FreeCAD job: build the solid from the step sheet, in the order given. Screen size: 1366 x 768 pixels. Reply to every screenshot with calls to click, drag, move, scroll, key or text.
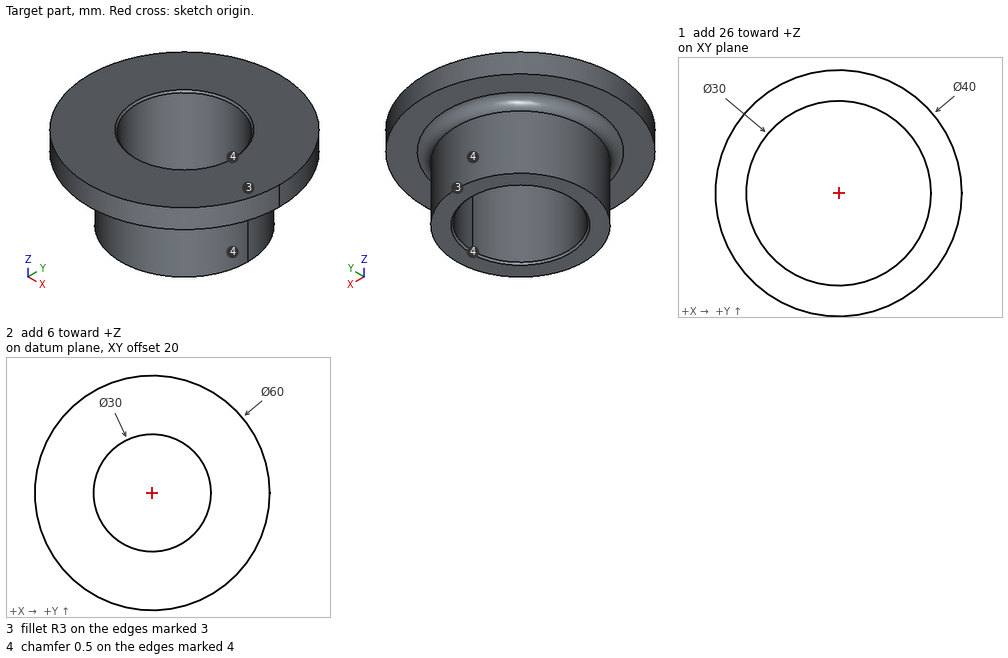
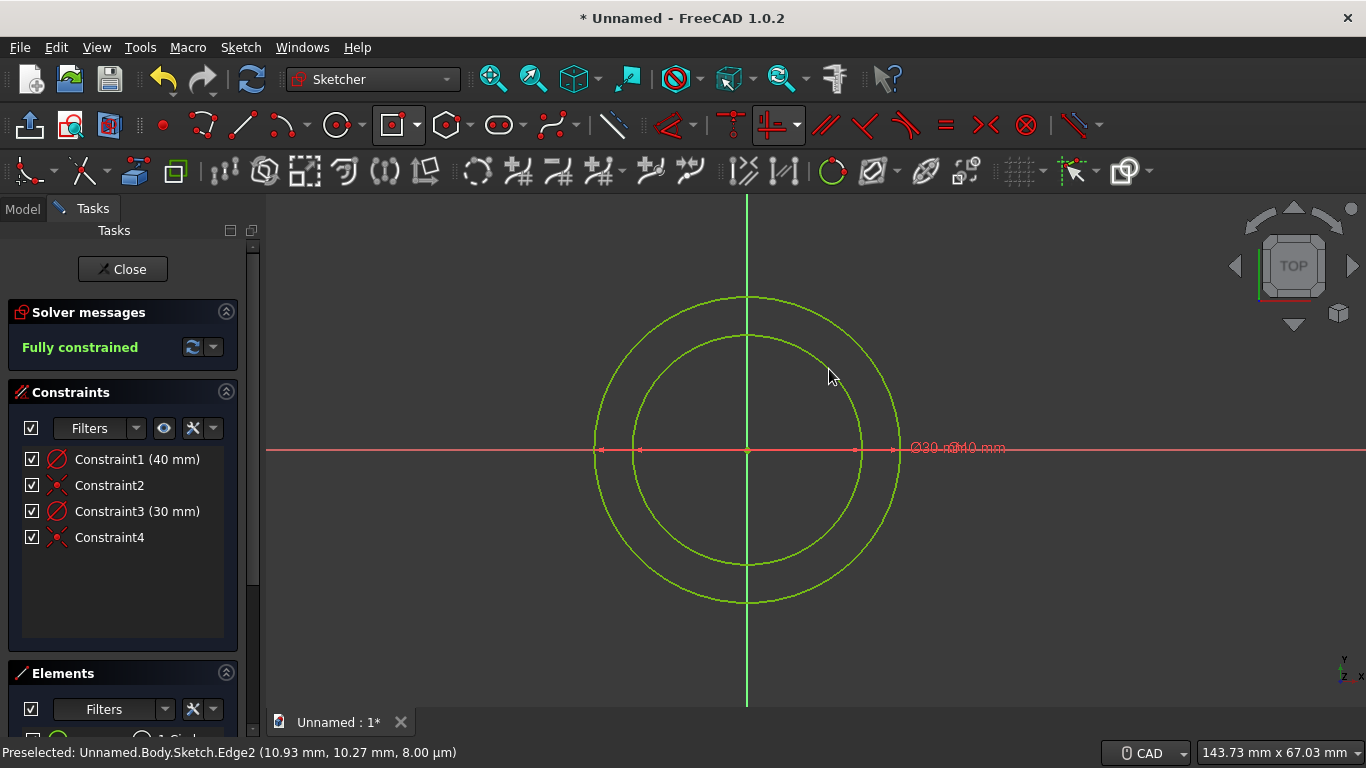
click(123, 269)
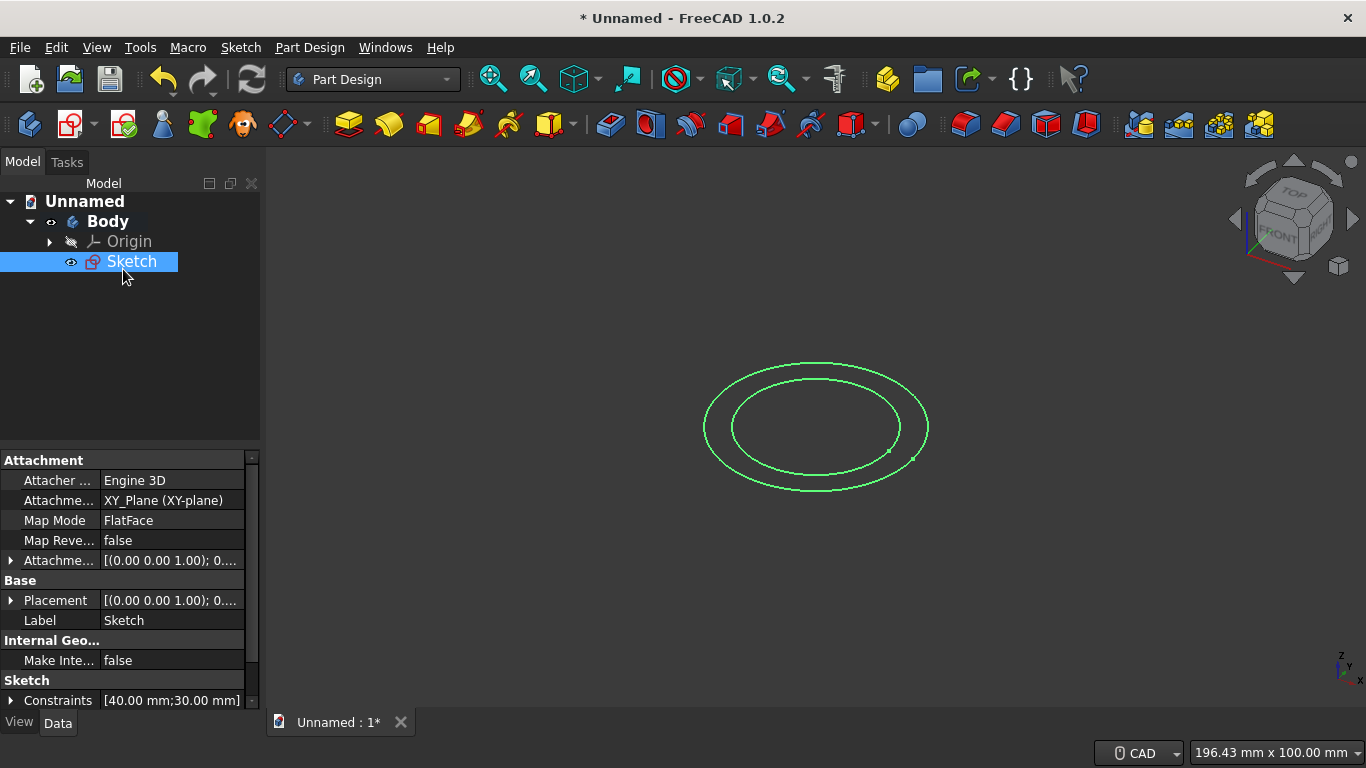
click(350, 124)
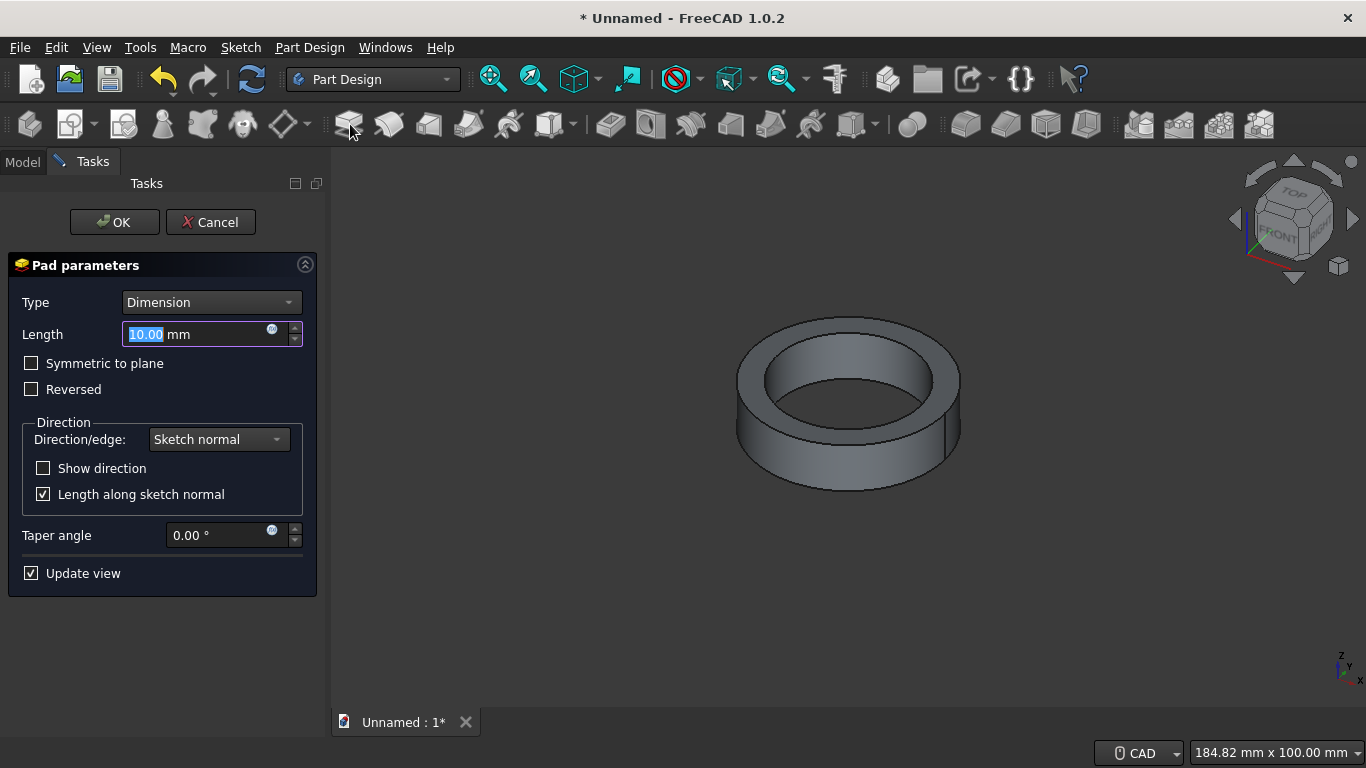
text(26)
key(Tab)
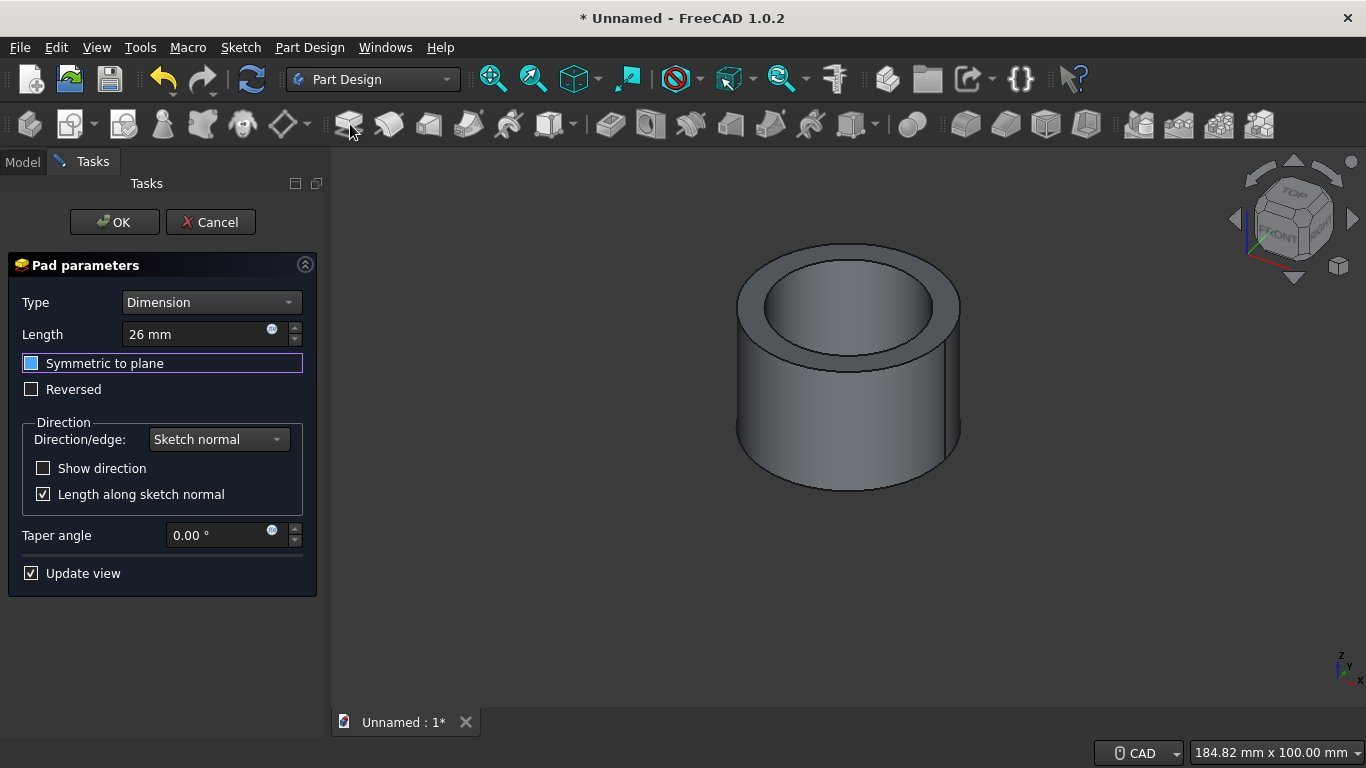
click(115, 222)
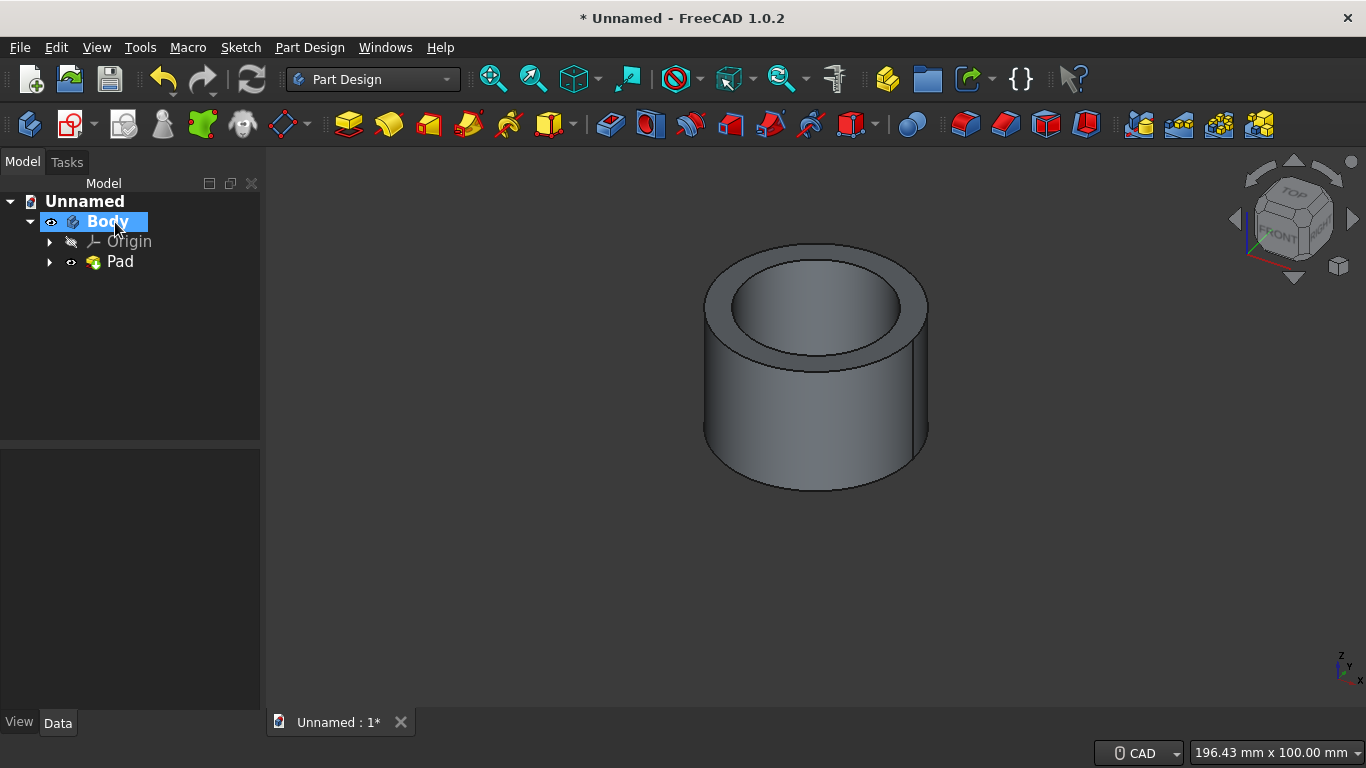
click(50, 242)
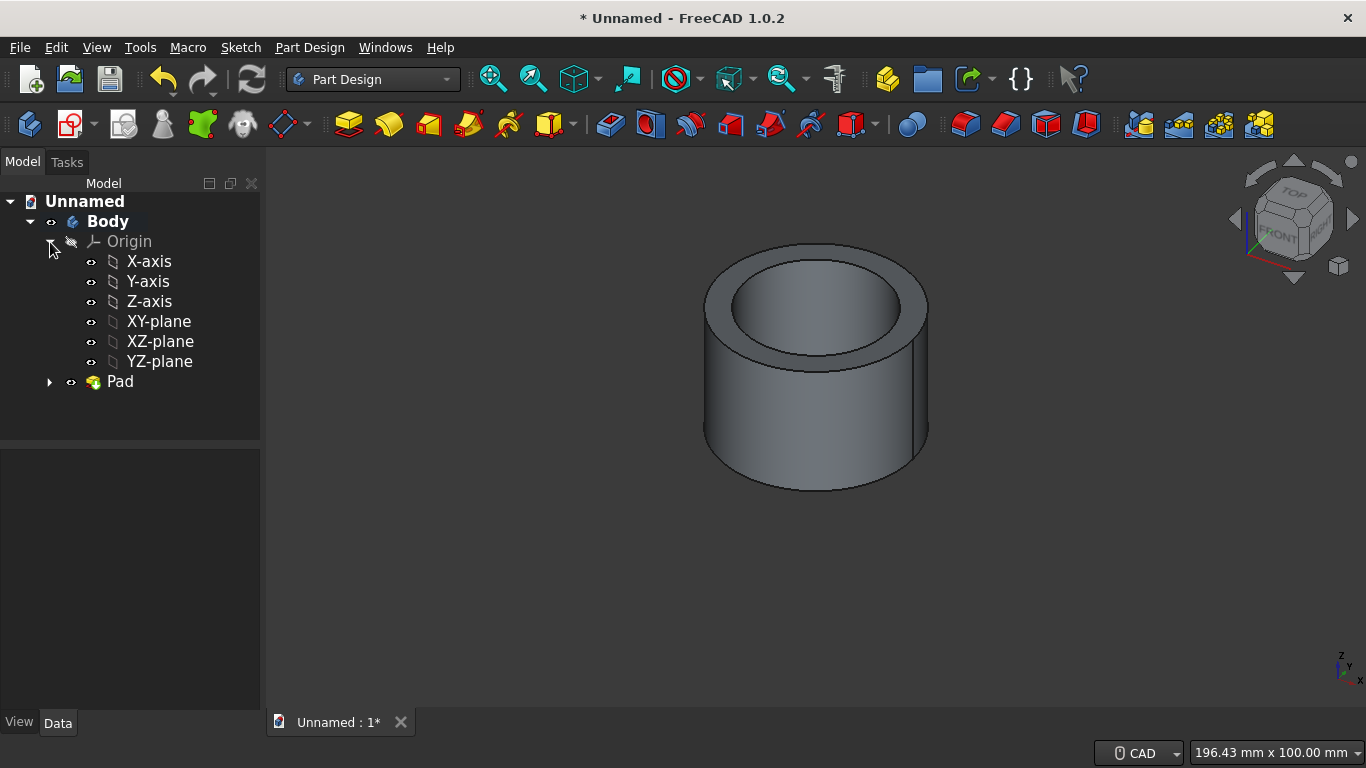
click(136, 322)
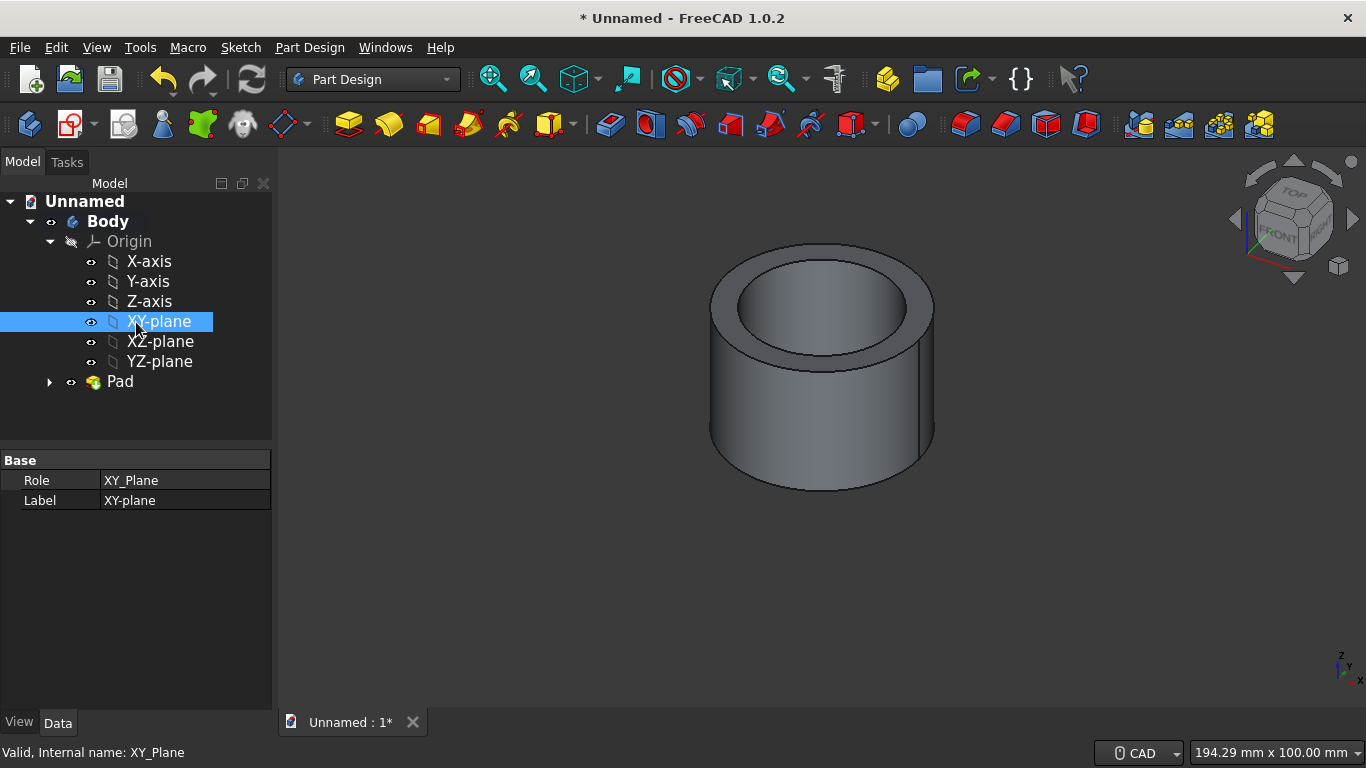
click(284, 124)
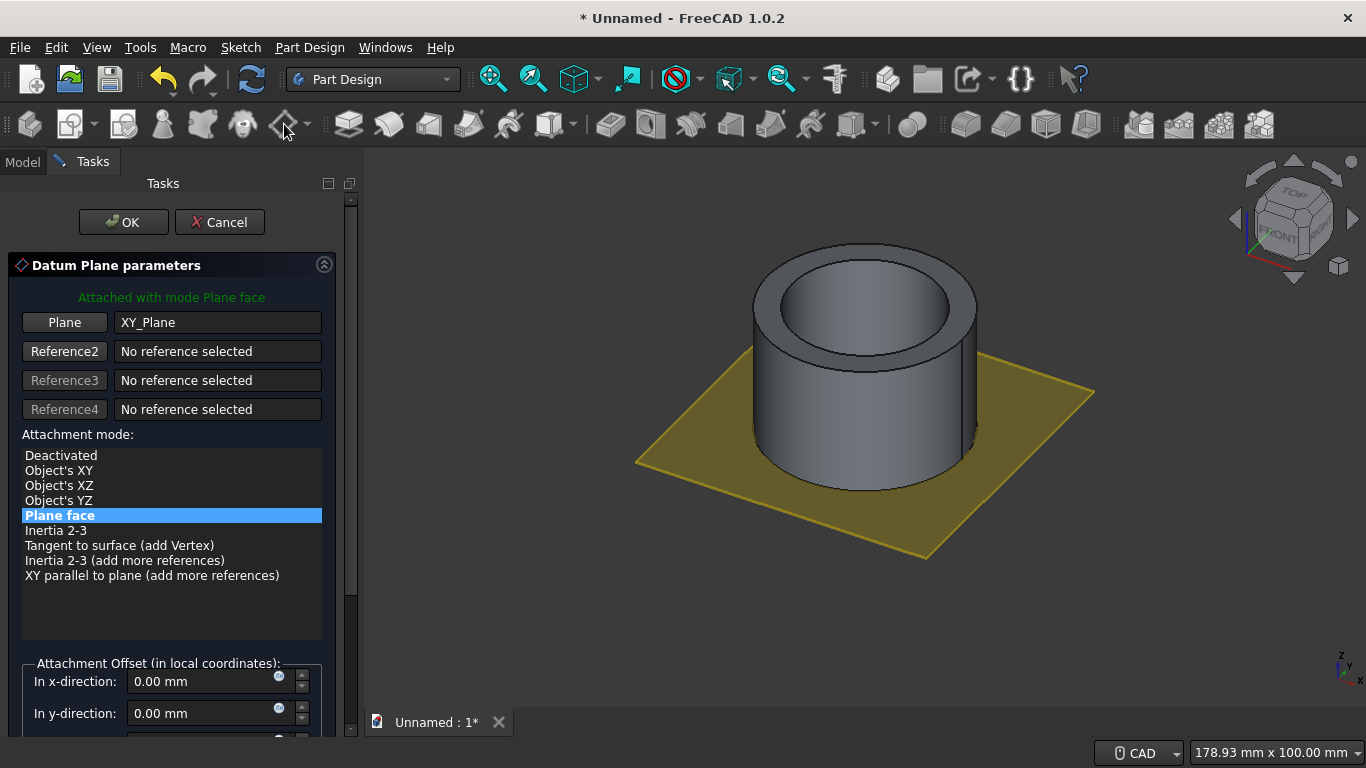
scroll(351, 464, down, 2)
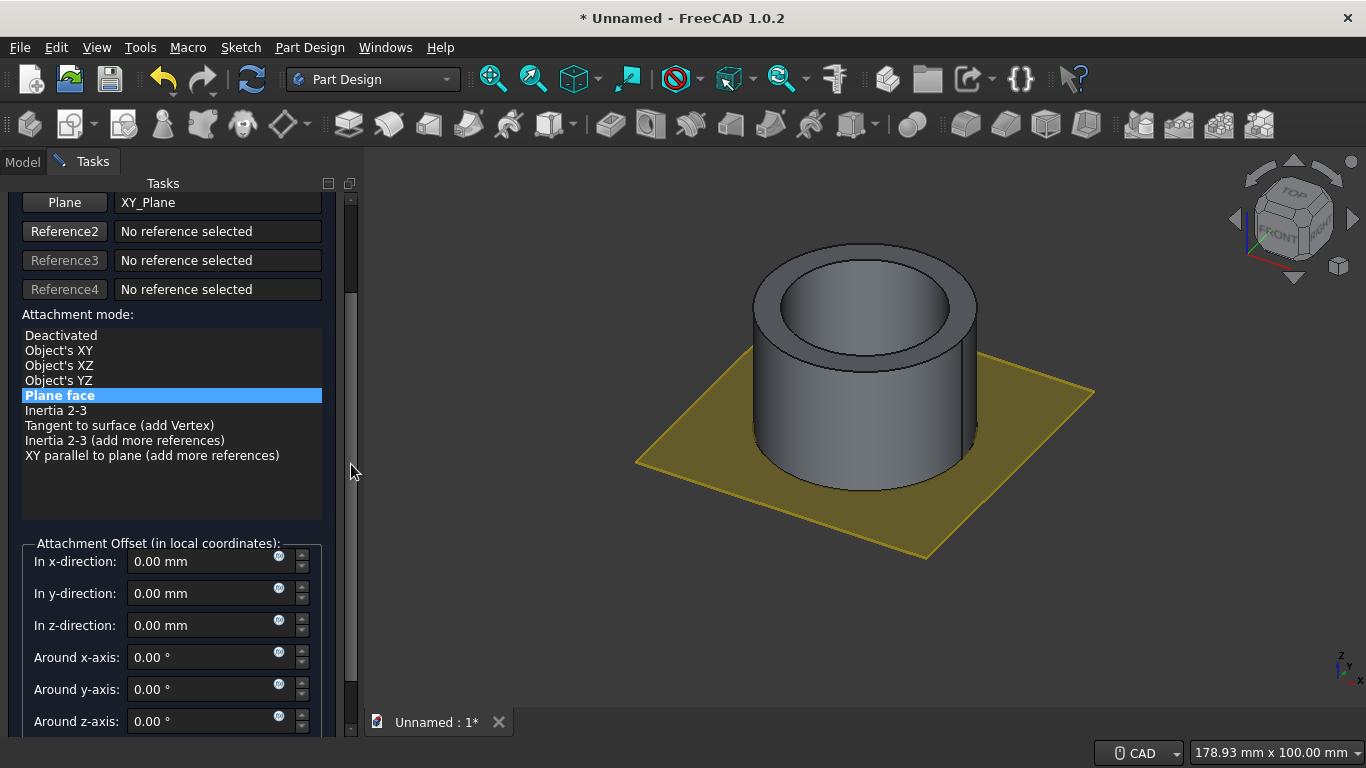
triple_click(210, 625)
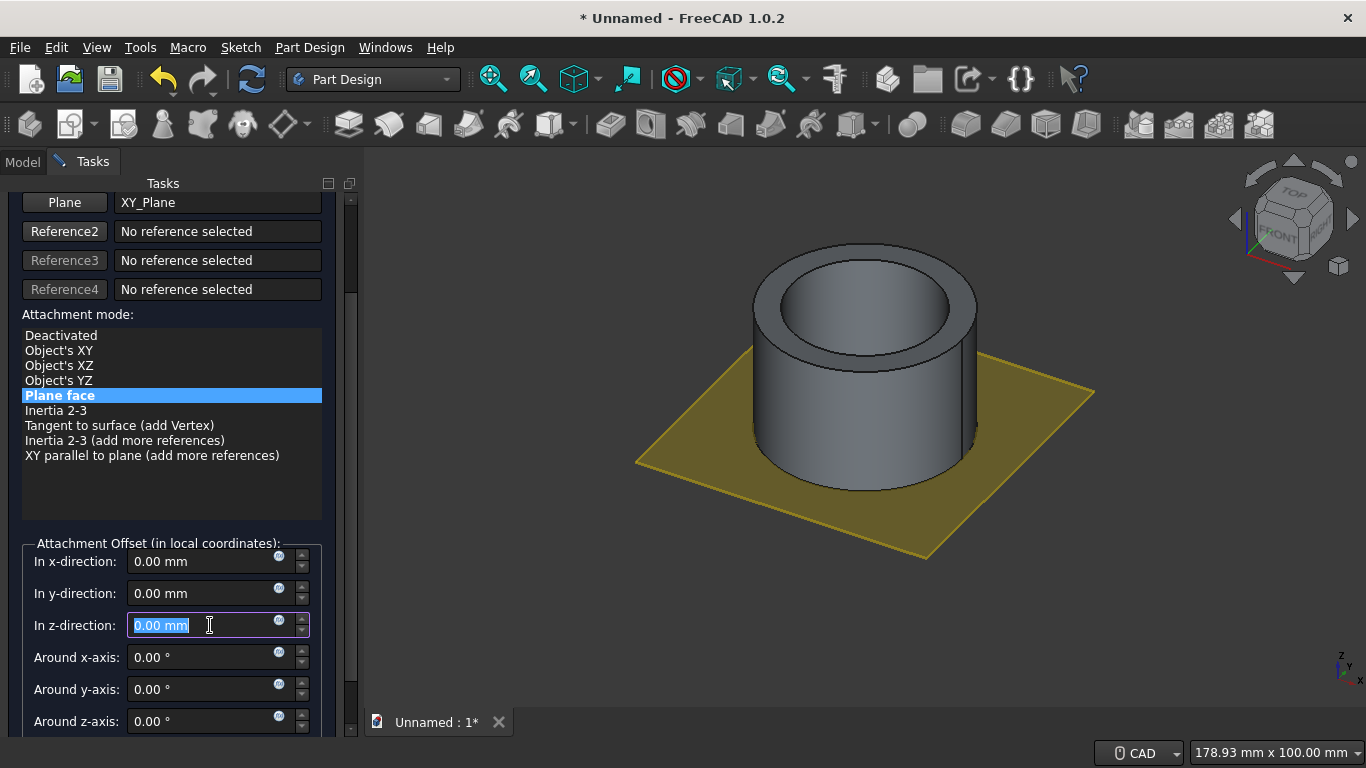
text(20)
key(Tab)